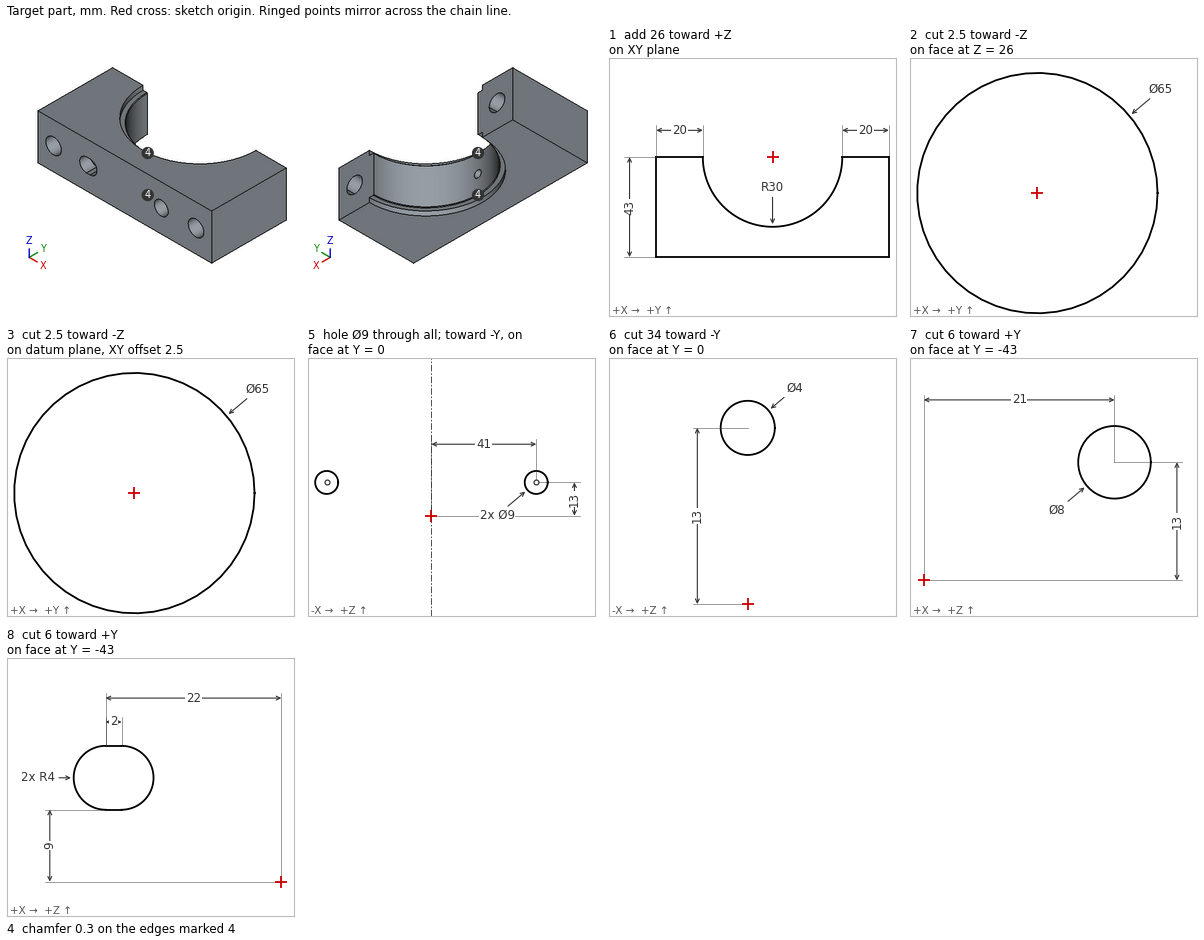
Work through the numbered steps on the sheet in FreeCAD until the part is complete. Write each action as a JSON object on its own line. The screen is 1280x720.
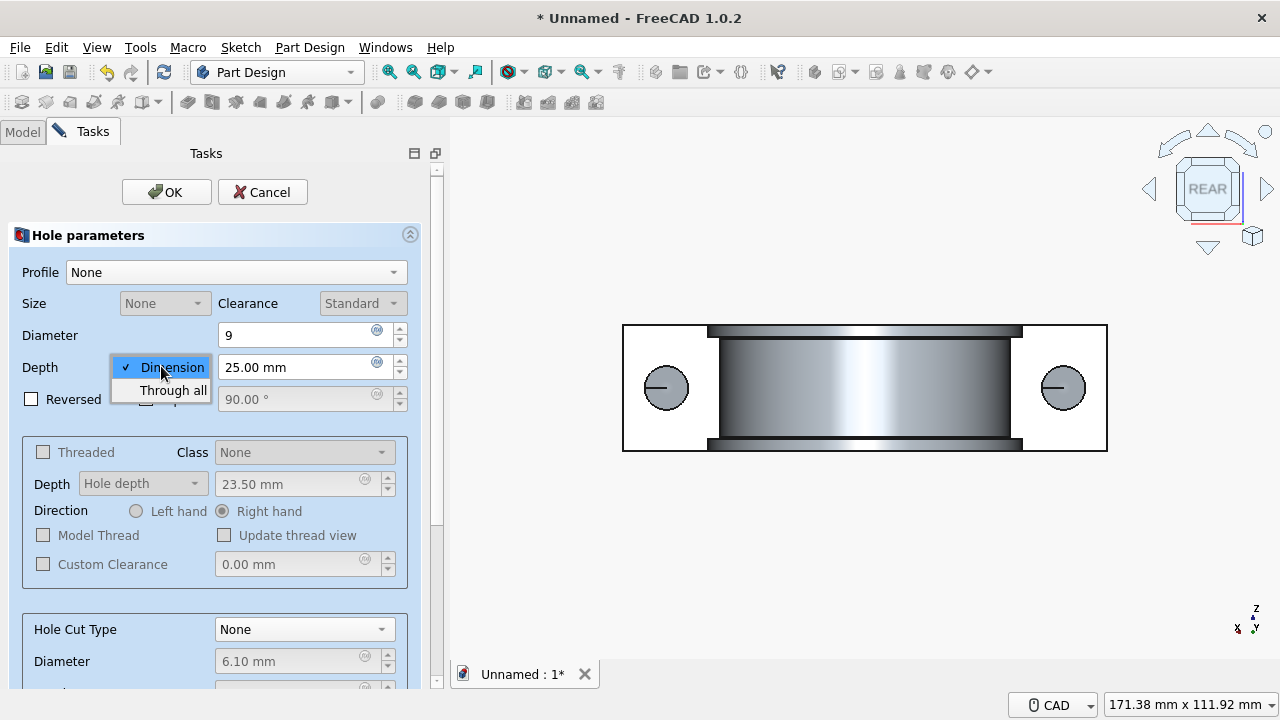
{"action": "left_click", "coordinate": [160, 390]}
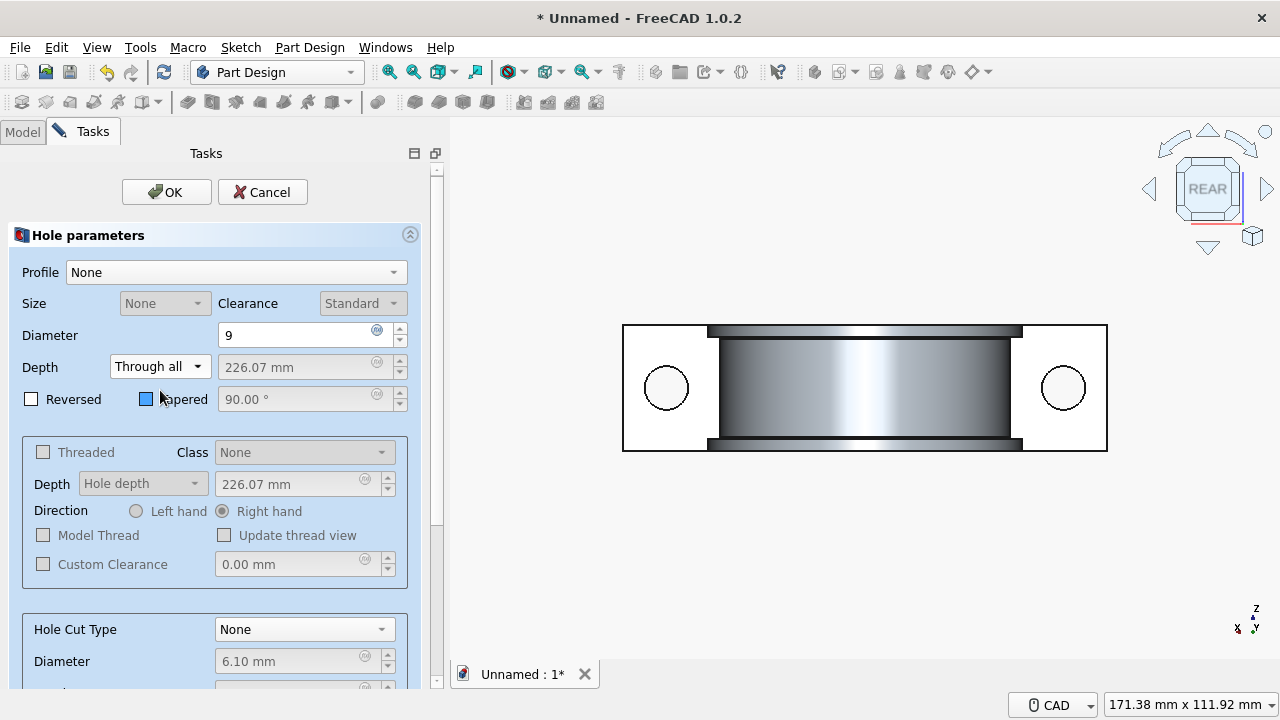
{"action": "left_click", "coordinate": [167, 192]}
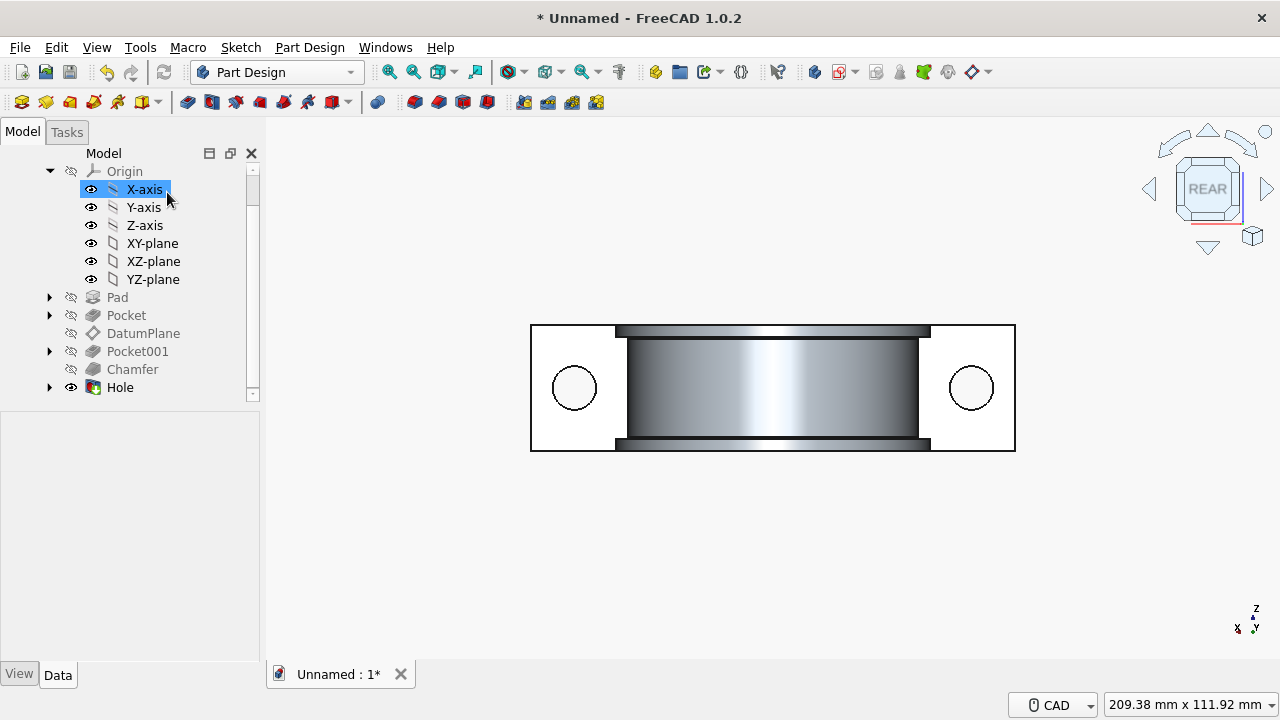
{"action": "left_click", "coordinate": [994, 351]}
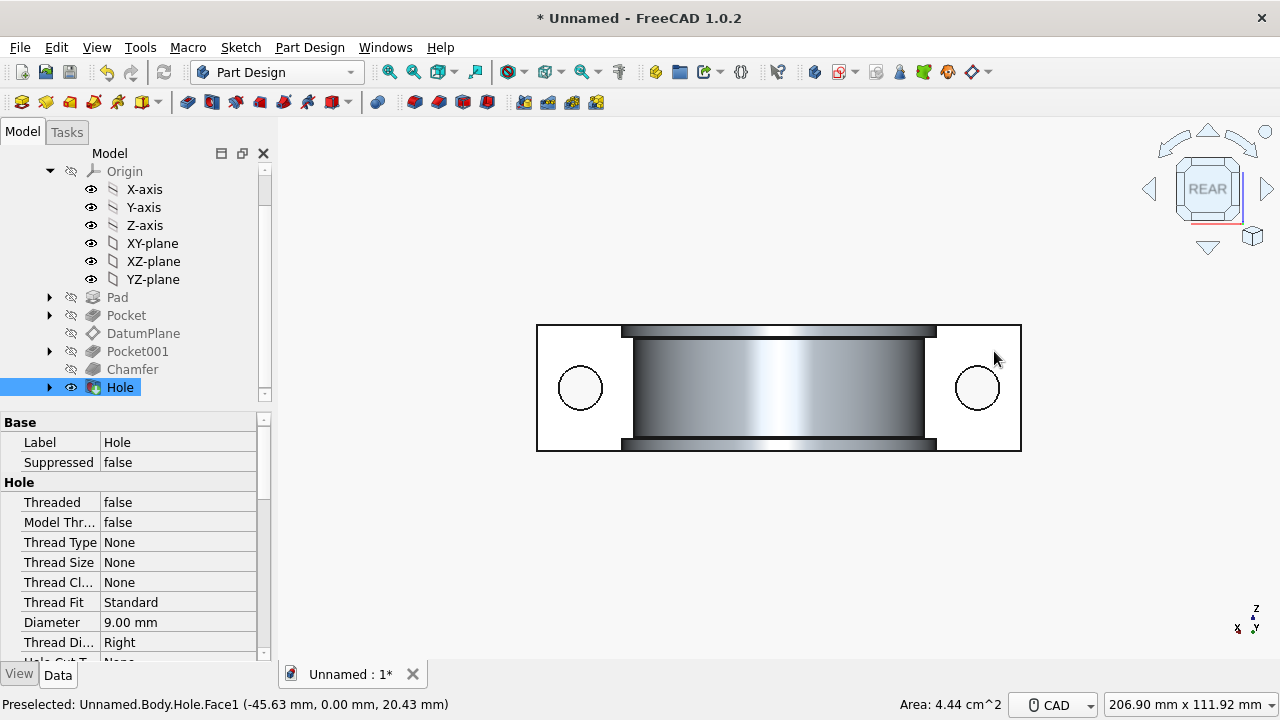
{"action": "left_click", "coordinate": [840, 72]}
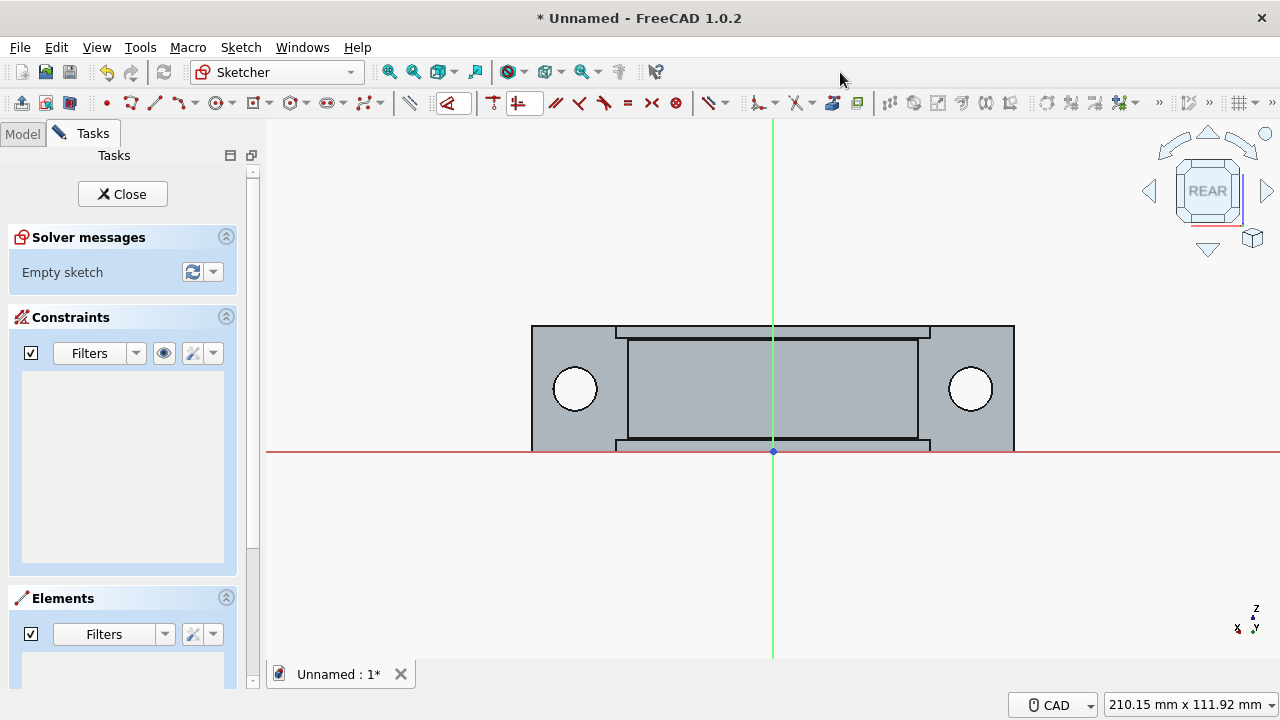
{"action": "scroll", "coordinate": [777, 389], "scroll_direction": "up", "scroll_amount": 14}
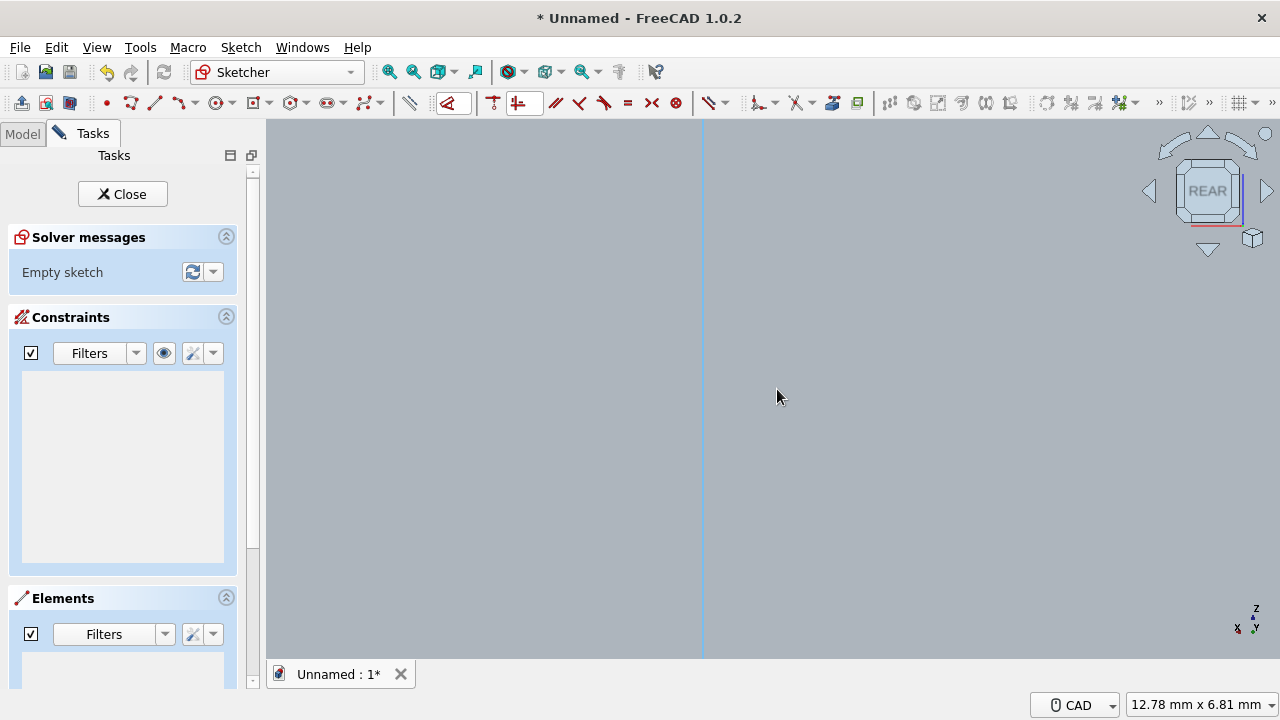
{"action": "left_click", "coordinate": [216, 104]}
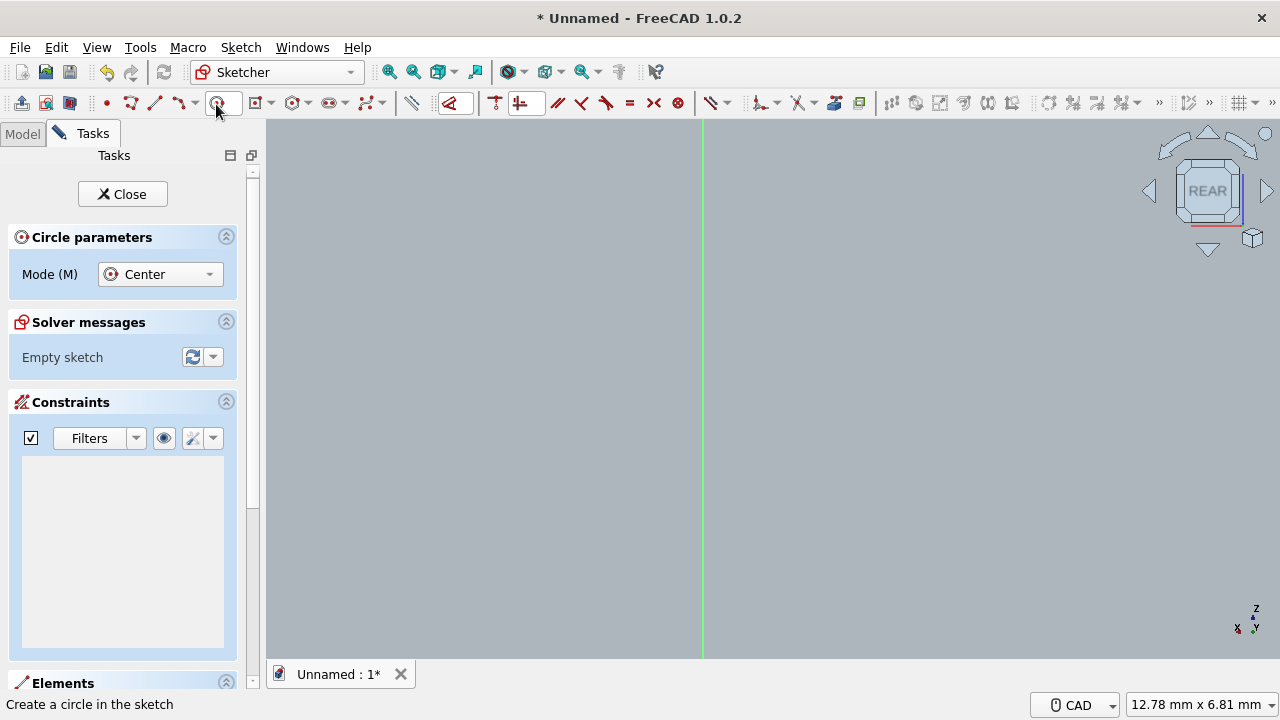
{"action": "left_click", "coordinate": [703, 381]}
{"action": "left_click", "coordinate": [816, 269]}
{"action": "key", "text": "Escape"}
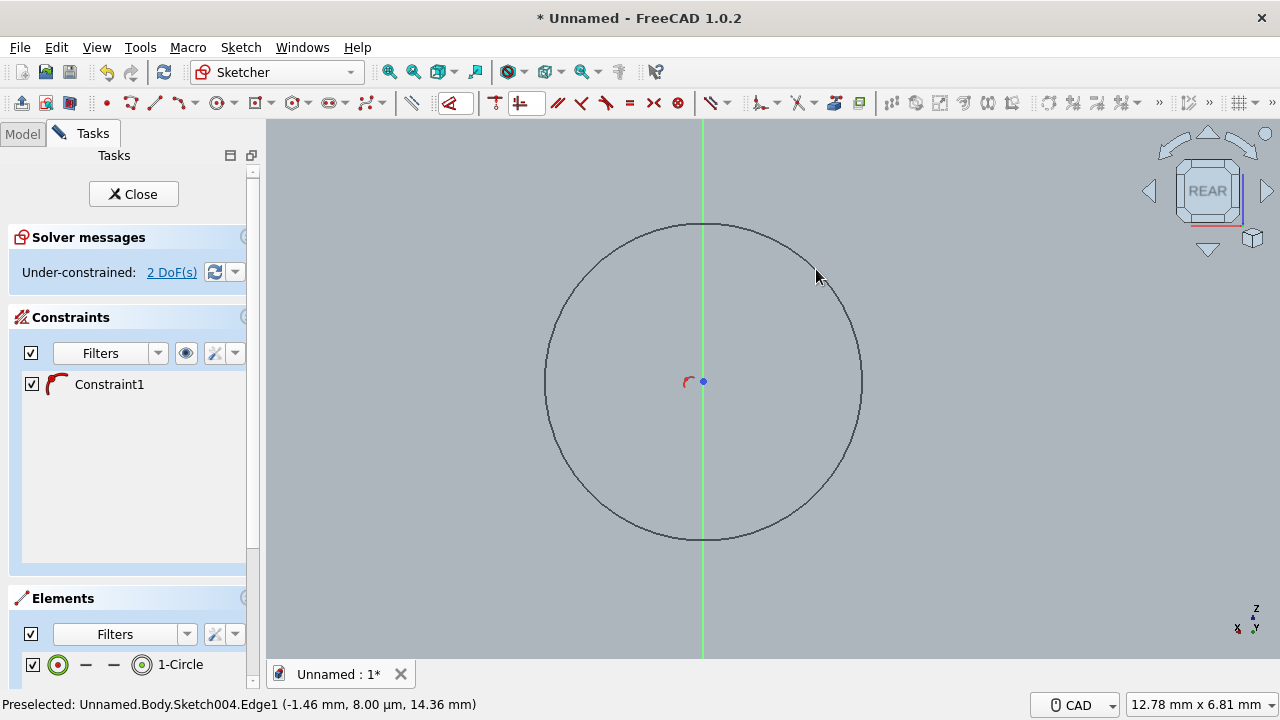
{"action": "left_click", "coordinate": [815, 269]}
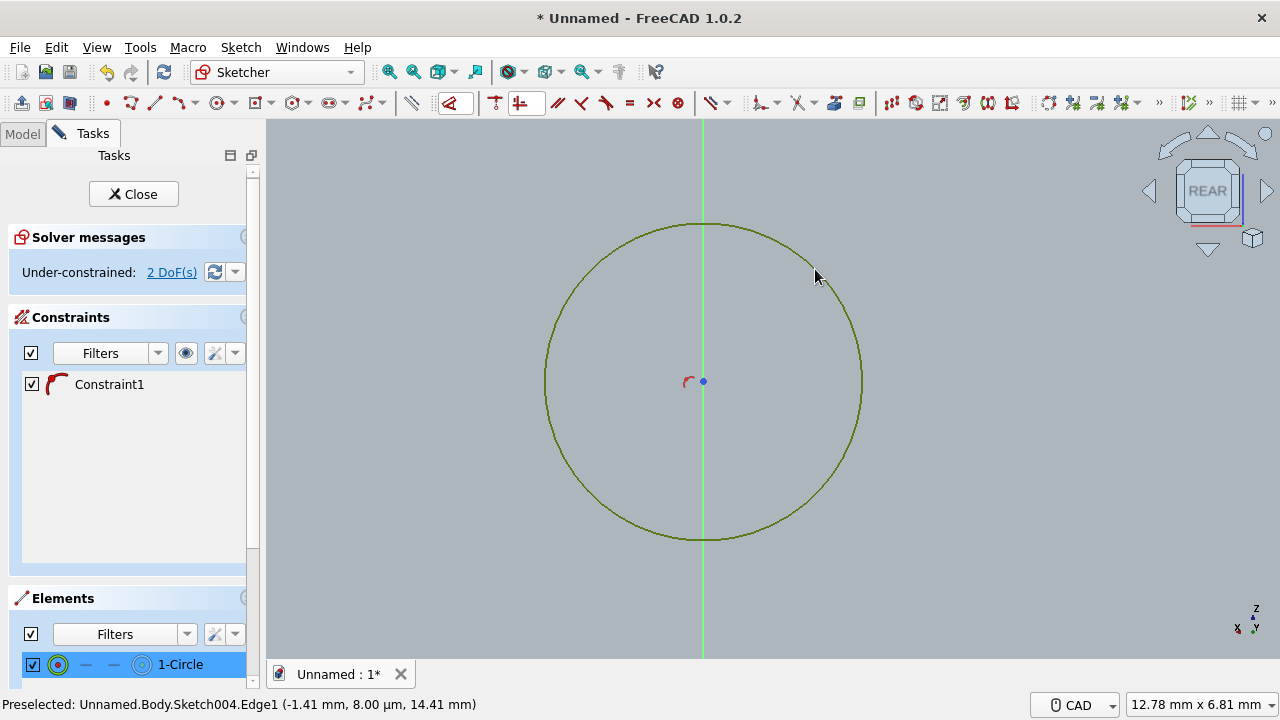
{"action": "left_click", "coordinate": [468, 104]}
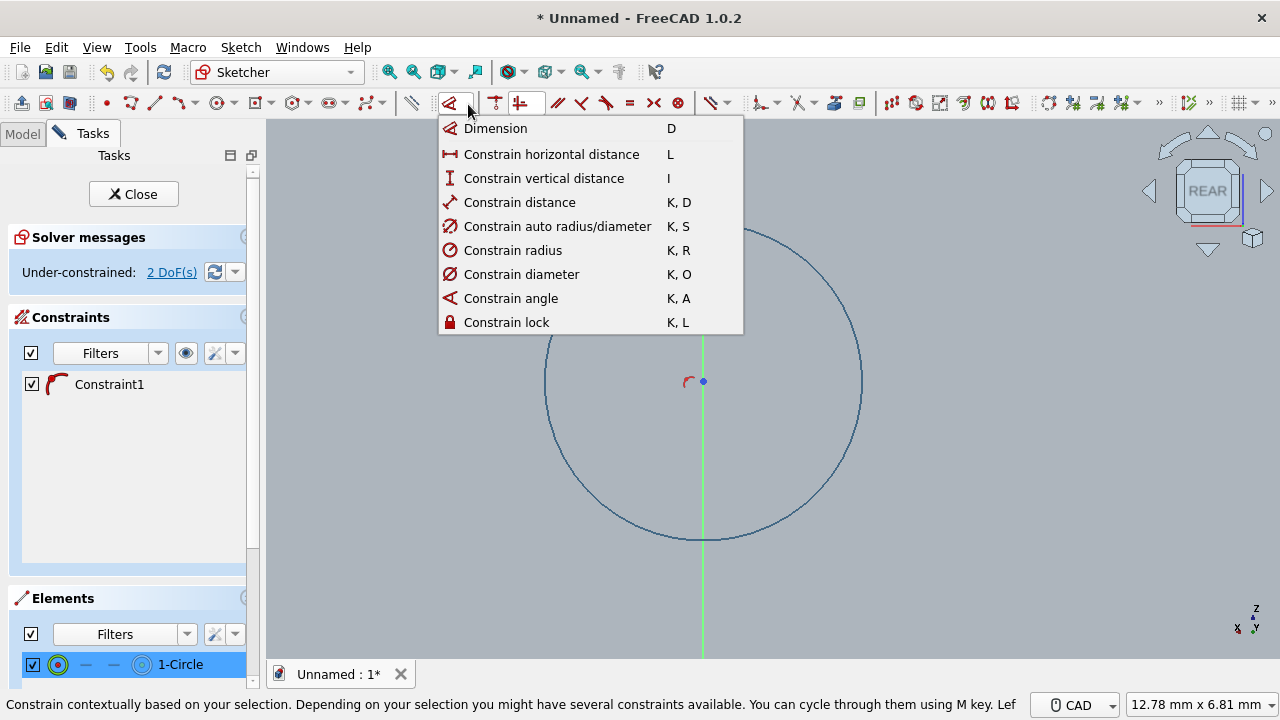
{"action": "left_click", "coordinate": [591, 274]}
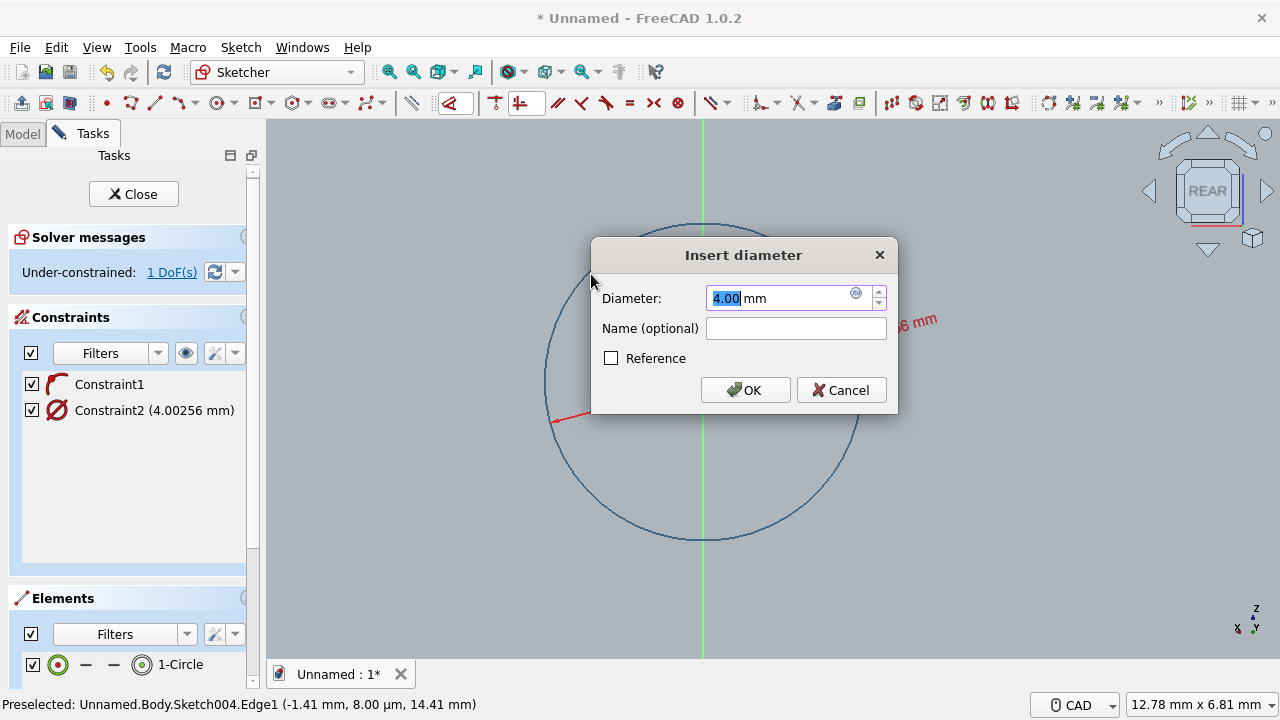
{"action": "type", "text": "4"}
{"action": "key", "text": "Return"}